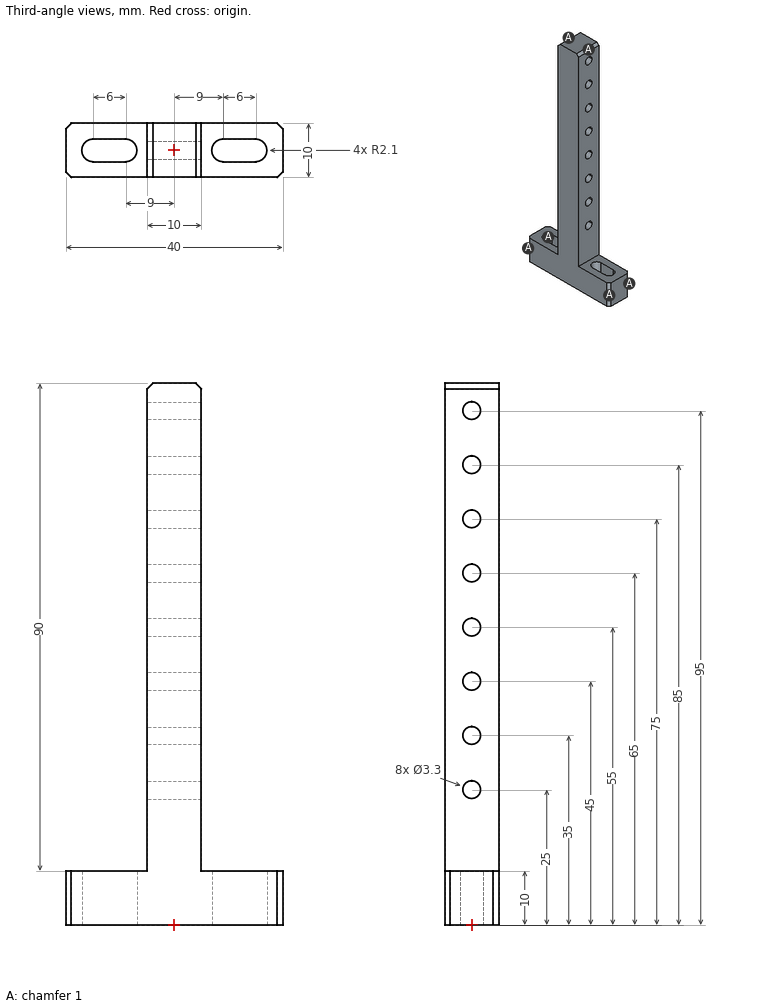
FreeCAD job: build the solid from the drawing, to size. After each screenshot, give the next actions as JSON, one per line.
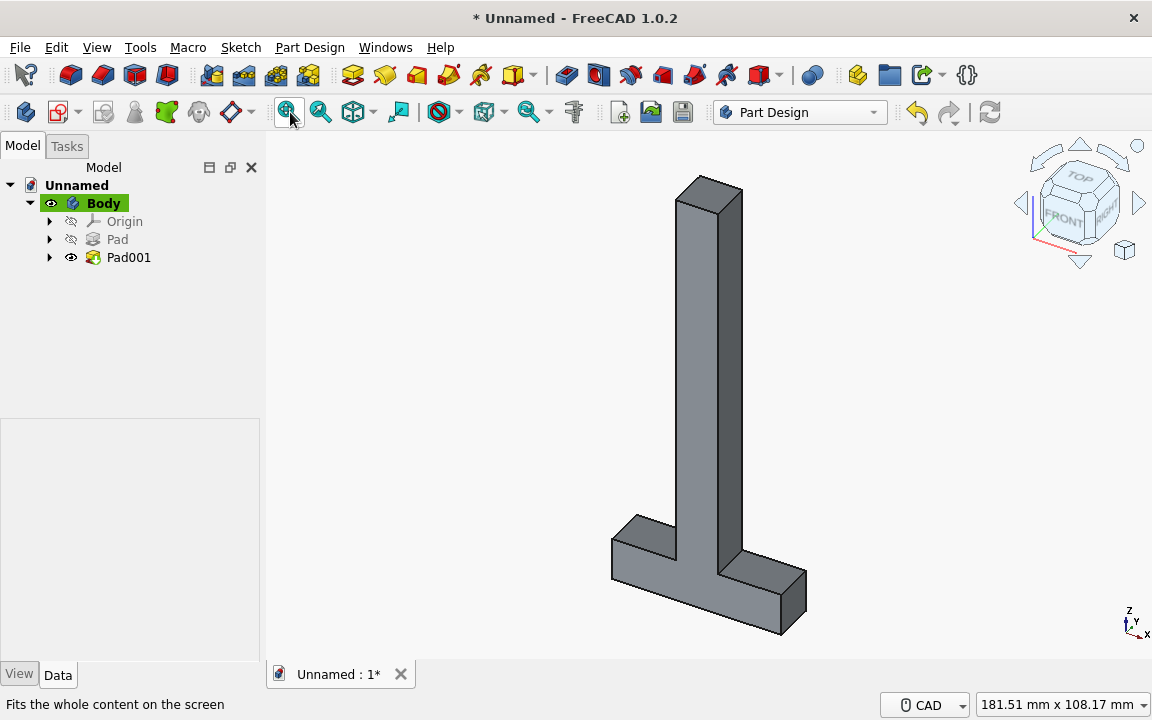
{"action": "left_click", "coordinate": [58, 112]}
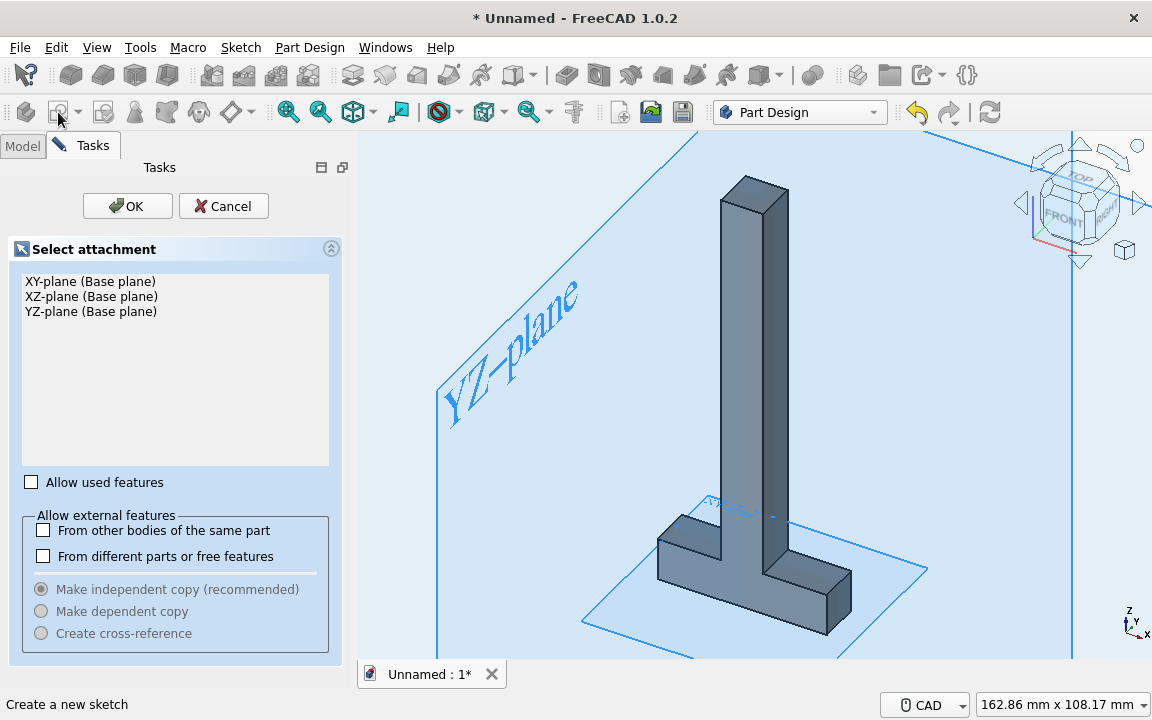
{"action": "left_click", "coordinate": [82, 282]}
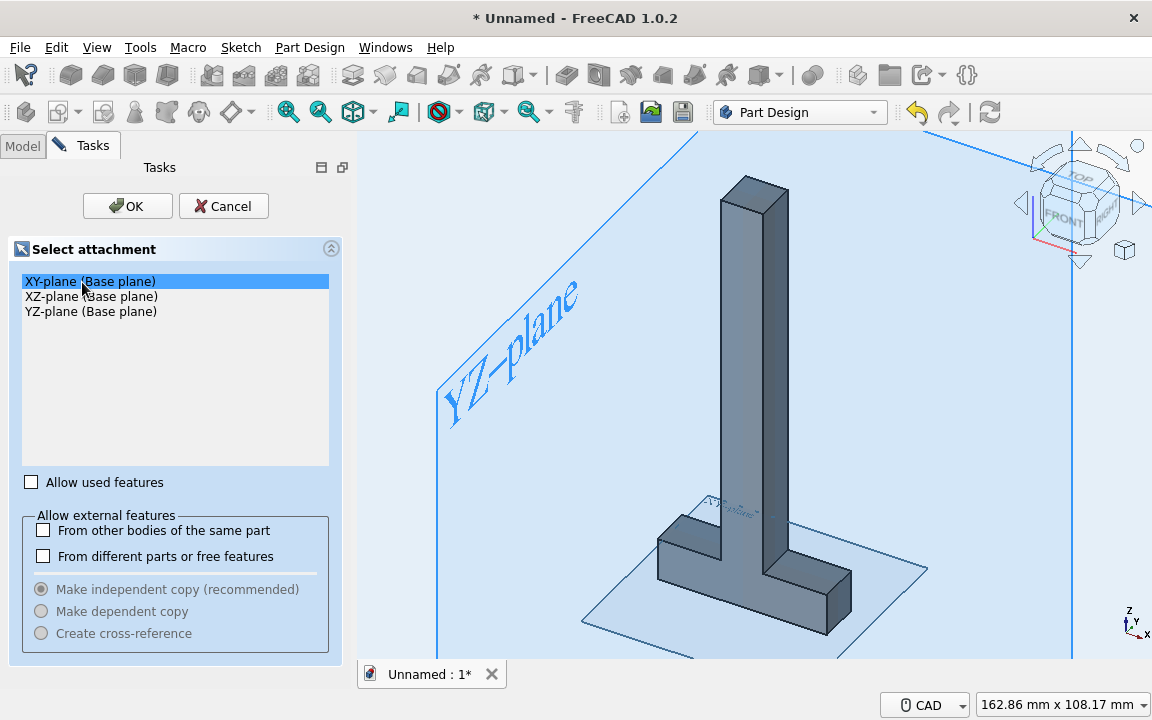
{"action": "left_click", "coordinate": [128, 206]}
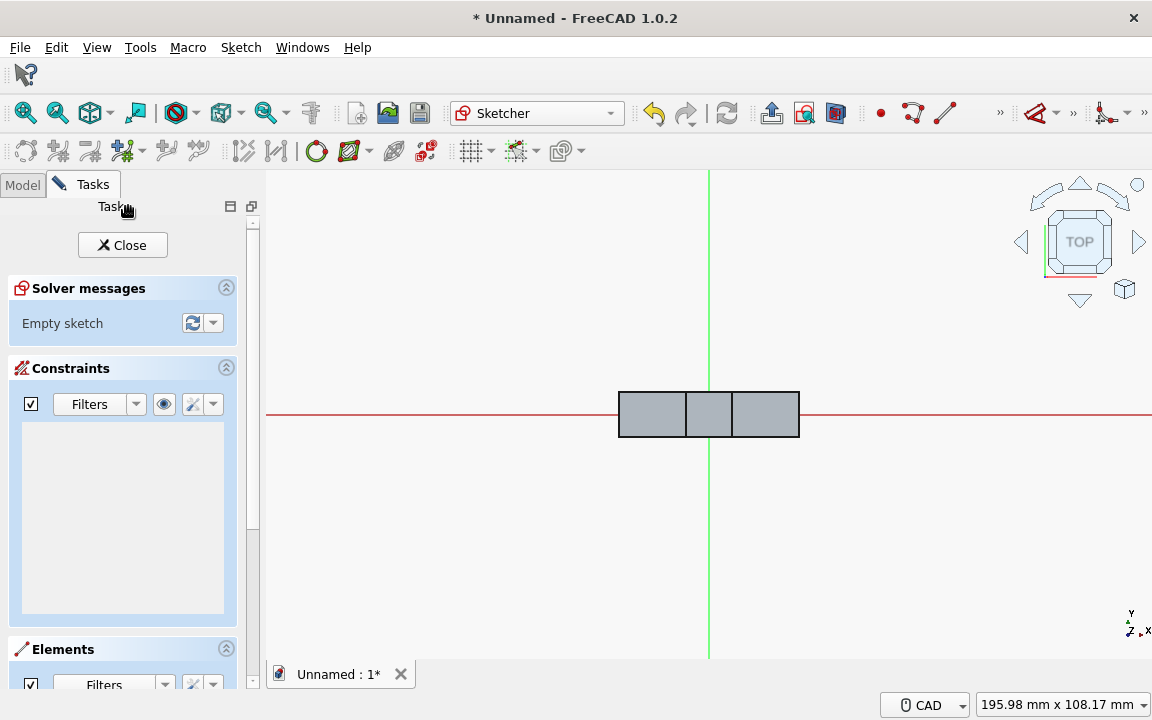
{"action": "left_click", "coordinate": [836, 114]}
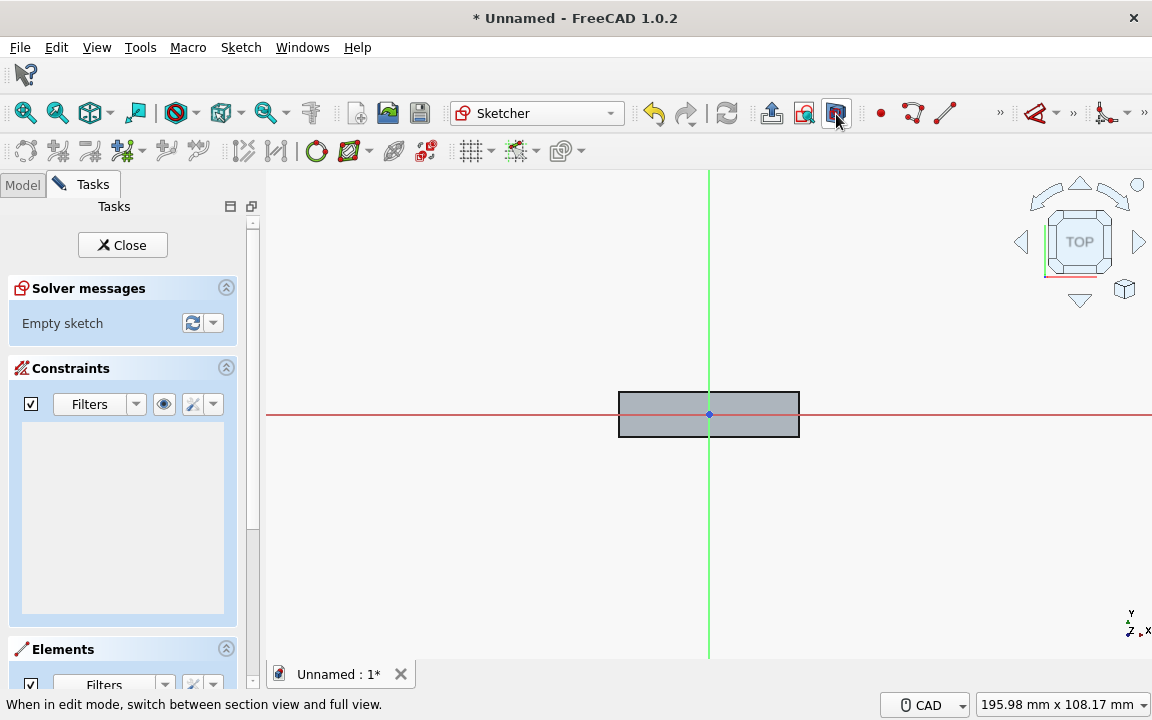
{"action": "scroll", "coordinate": [739, 415], "scroll_direction": "up", "scroll_amount": 6}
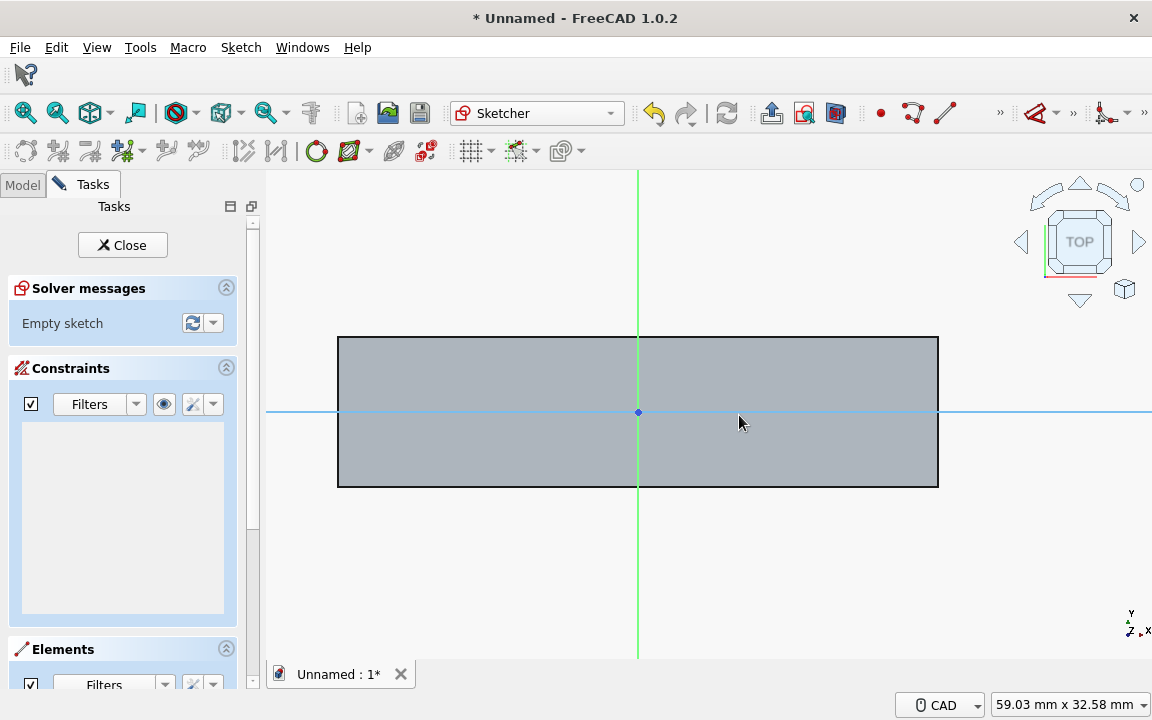
{"action": "key", "text": "g s"}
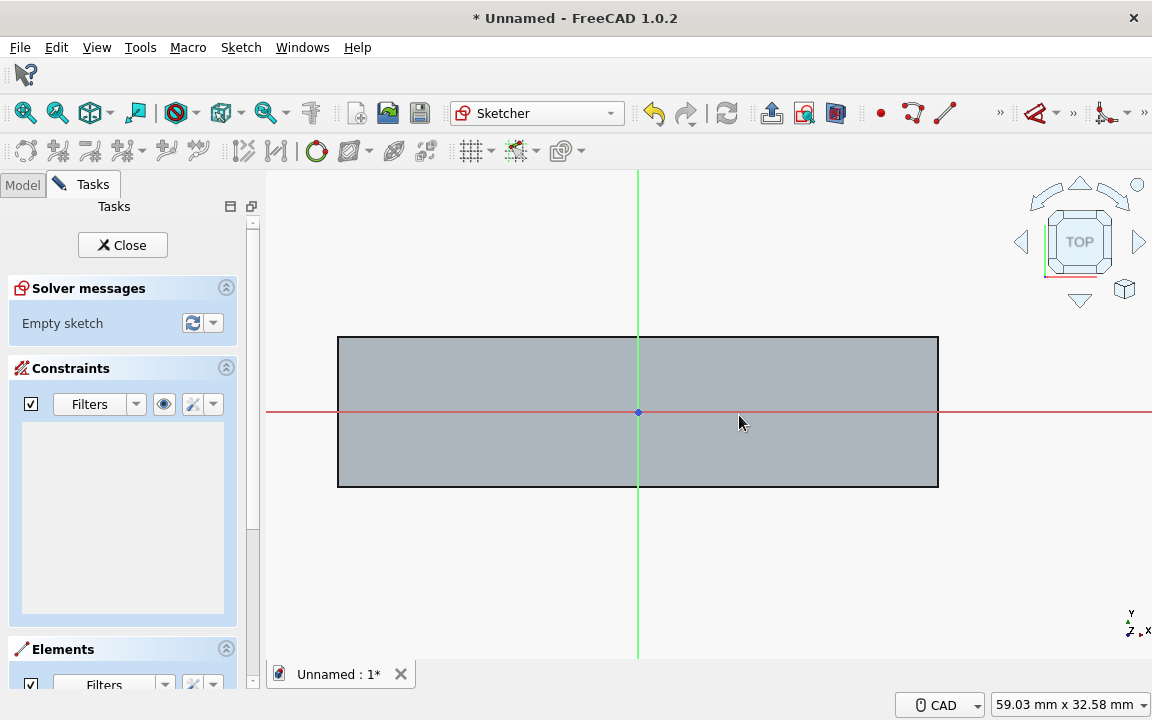
{"action": "left_click", "coordinate": [773, 412]}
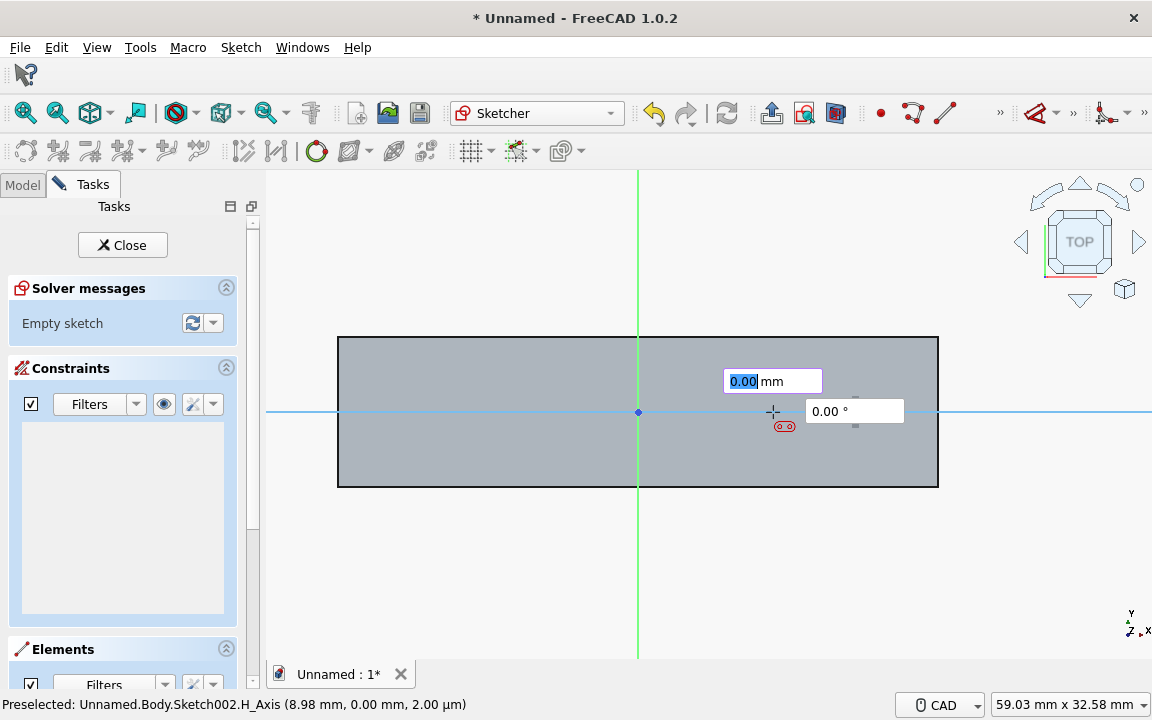
{"action": "left_click", "coordinate": [863, 403]}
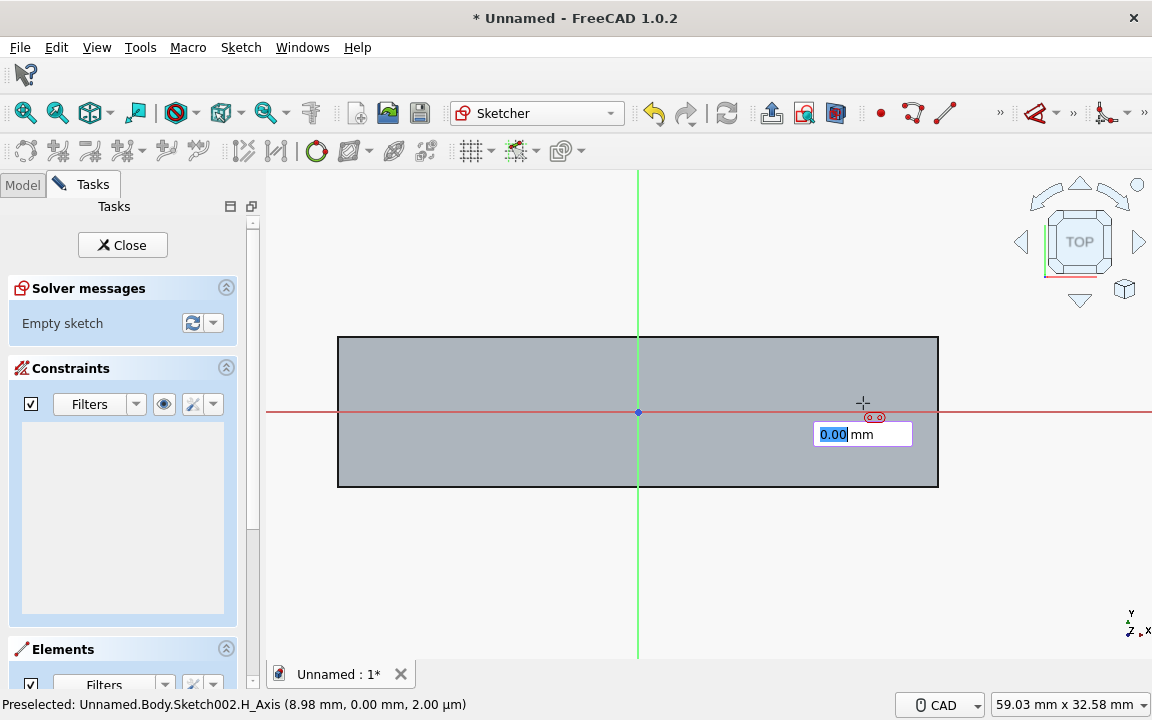
{"action": "left_click", "coordinate": [818, 381]}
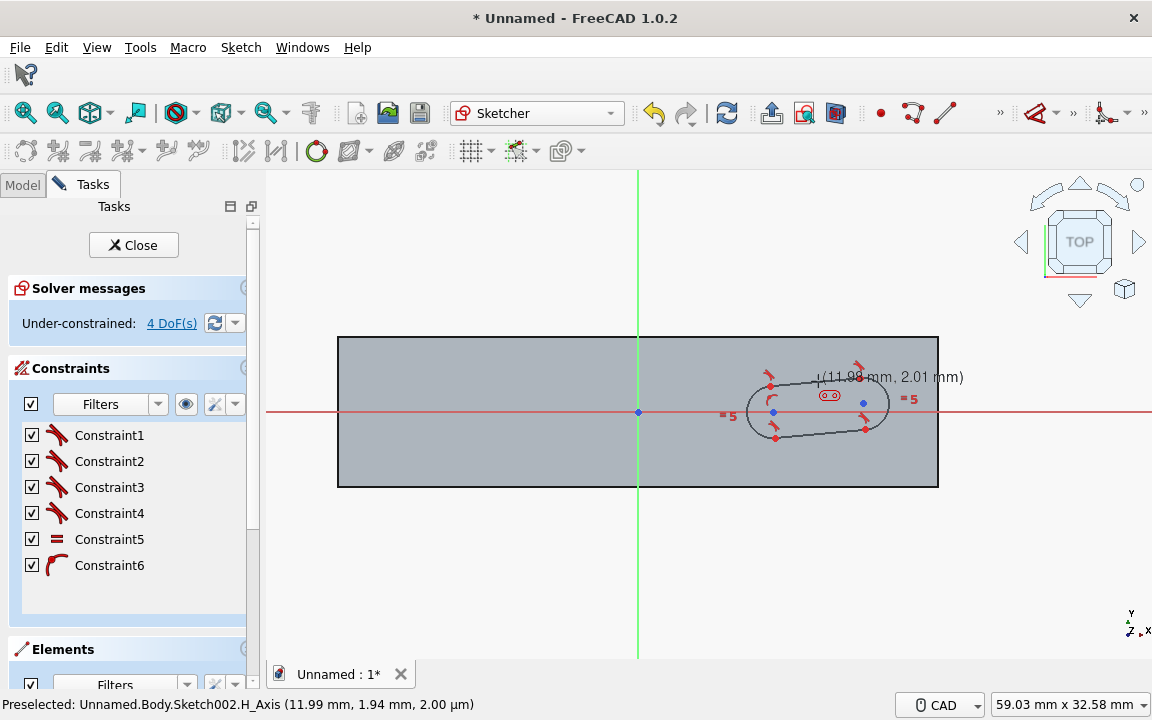
{"action": "left_click", "coordinate": [413, 412]}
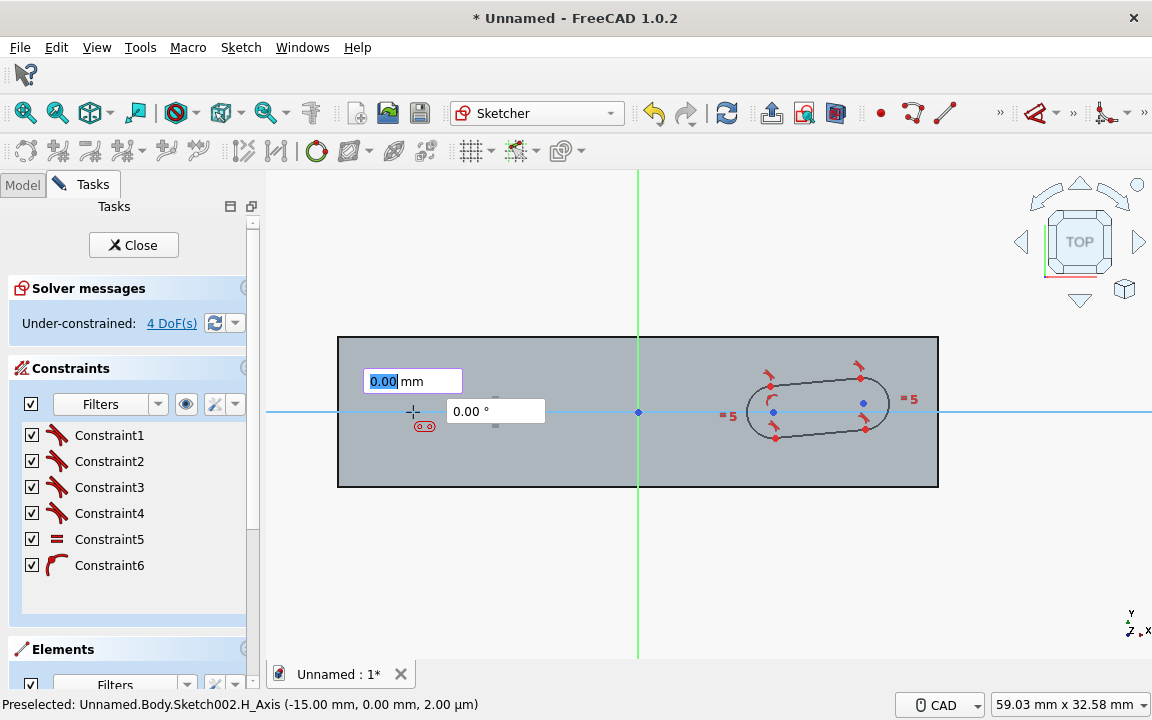
{"action": "left_click", "coordinate": [503, 403]}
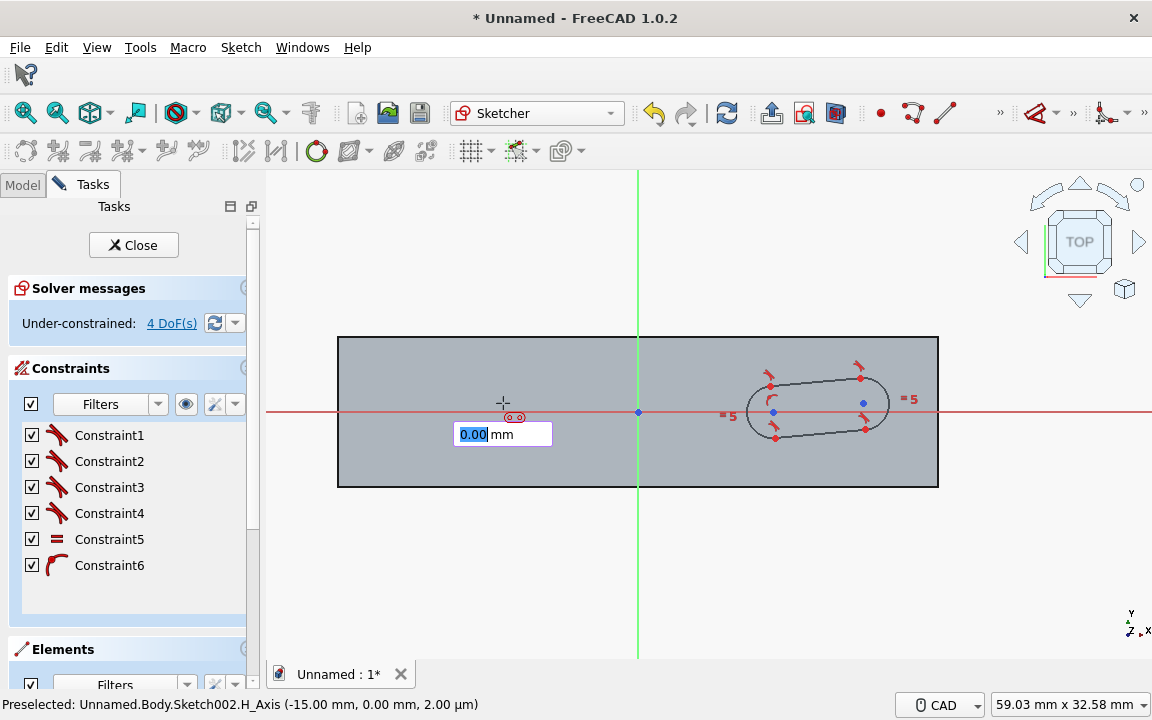
{"action": "left_click", "coordinate": [458, 381]}
{"action": "key", "text": "Escape"}